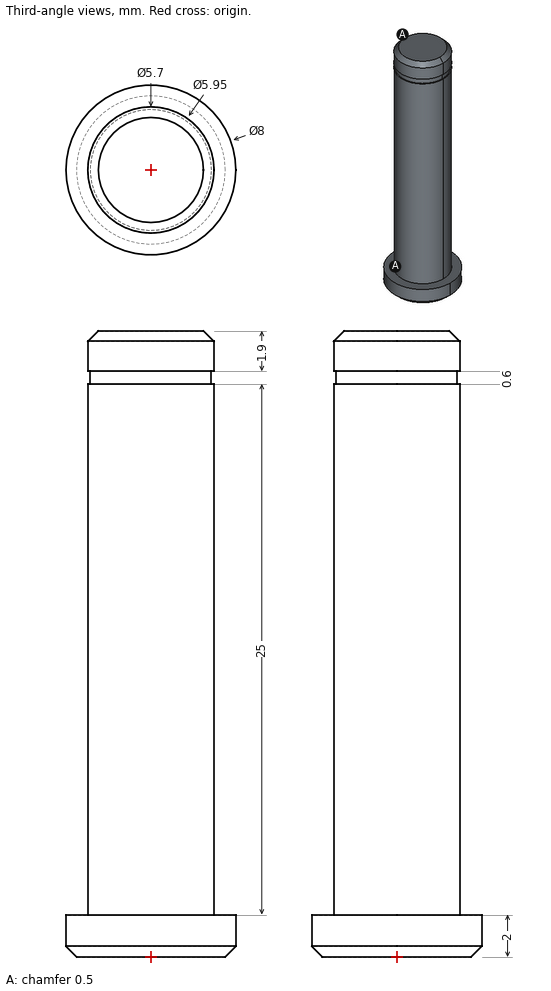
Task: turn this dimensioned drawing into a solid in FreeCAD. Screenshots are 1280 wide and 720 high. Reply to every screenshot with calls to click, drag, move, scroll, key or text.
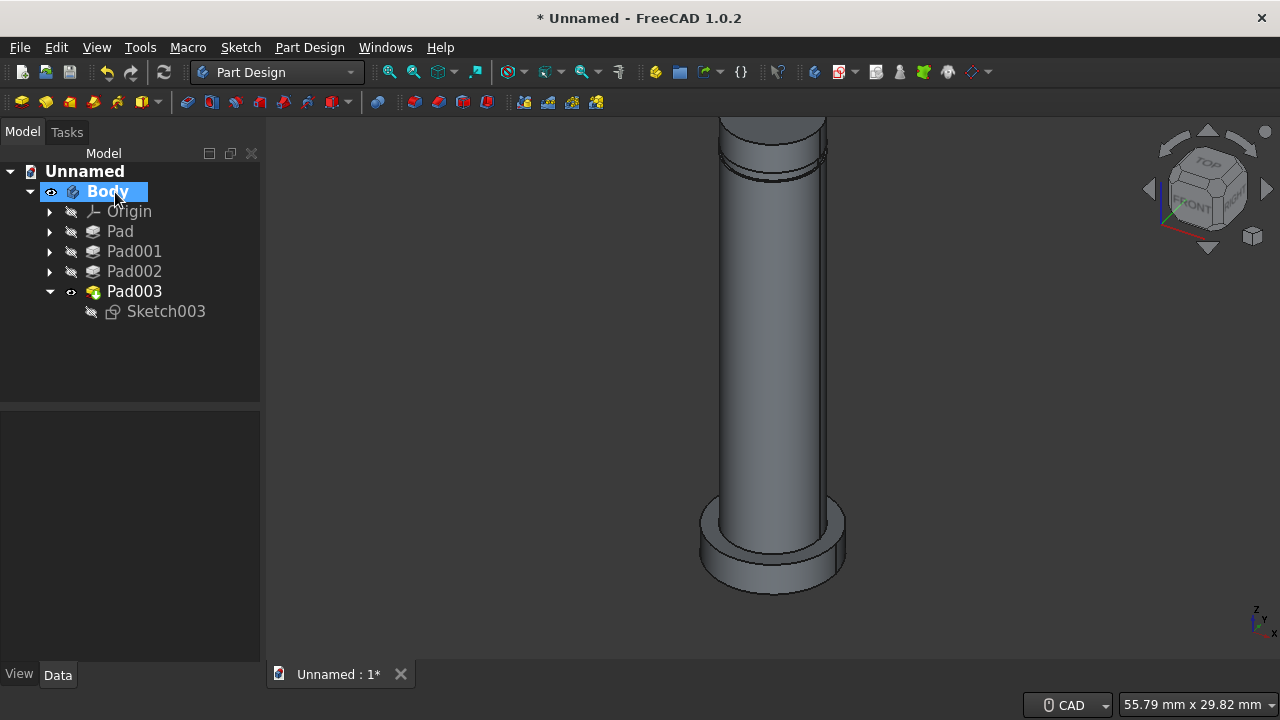
key(v)
key(f)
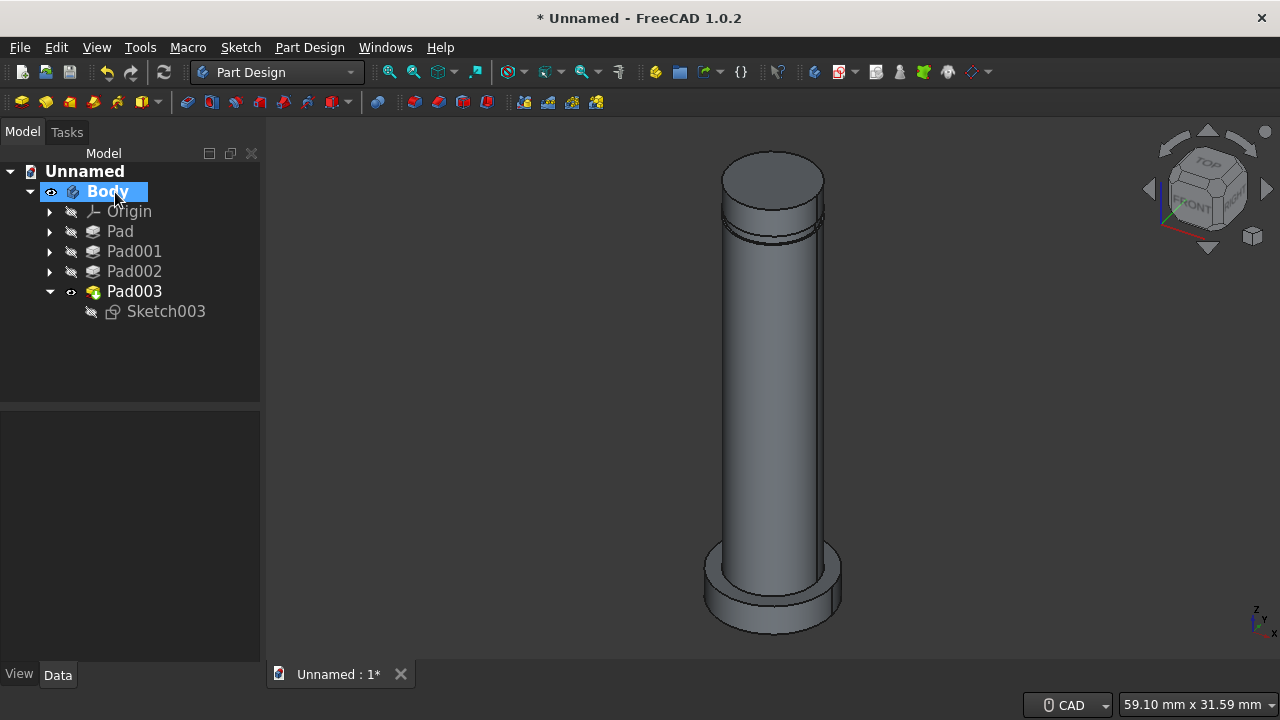
click(722, 183)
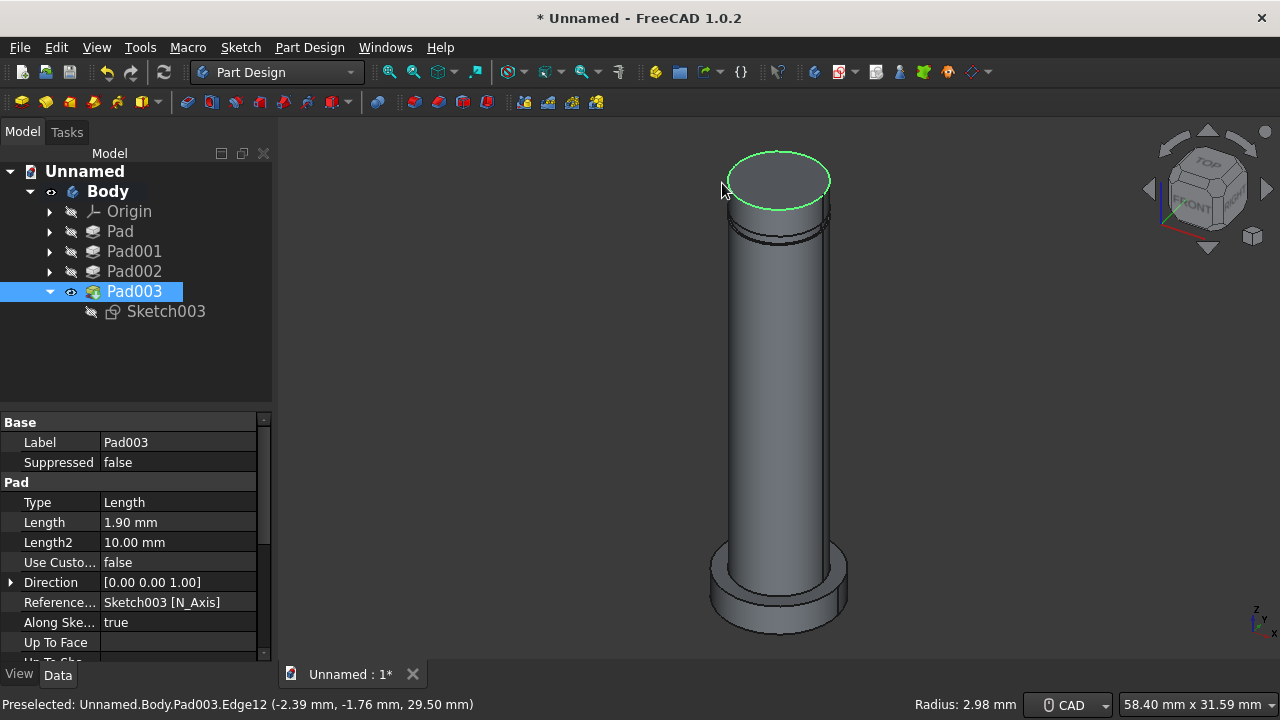
key(0)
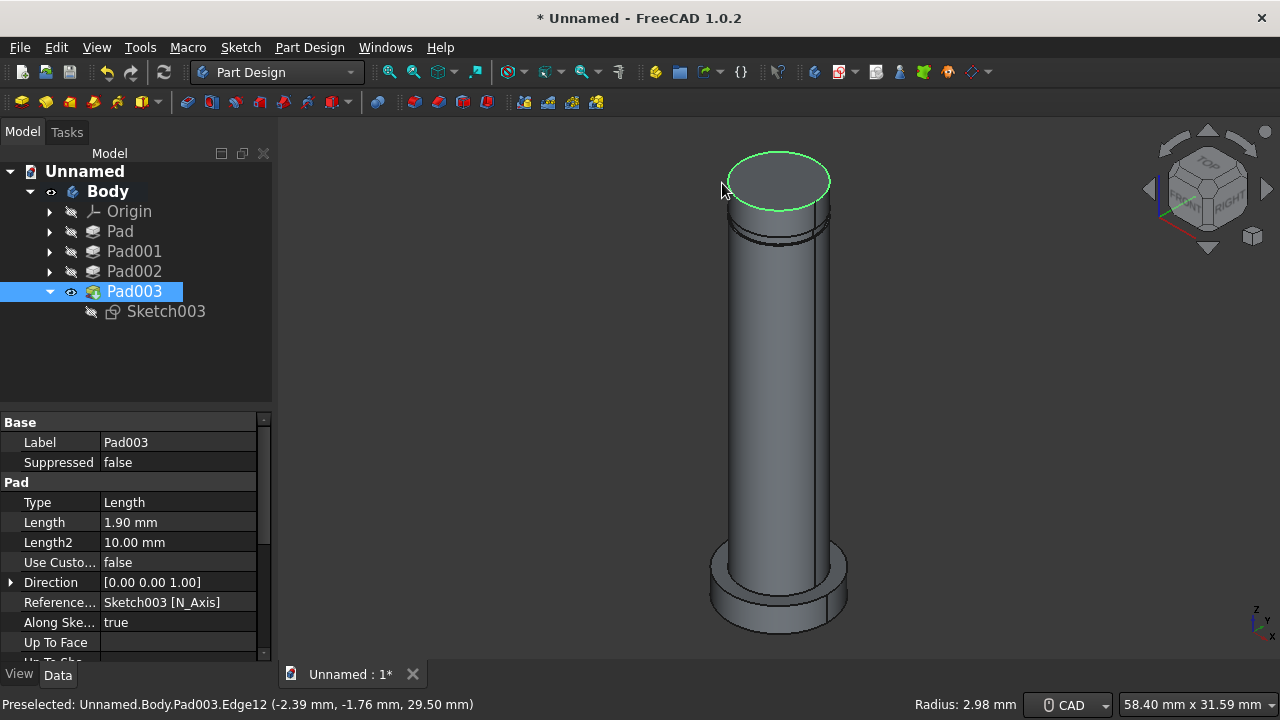
key(2)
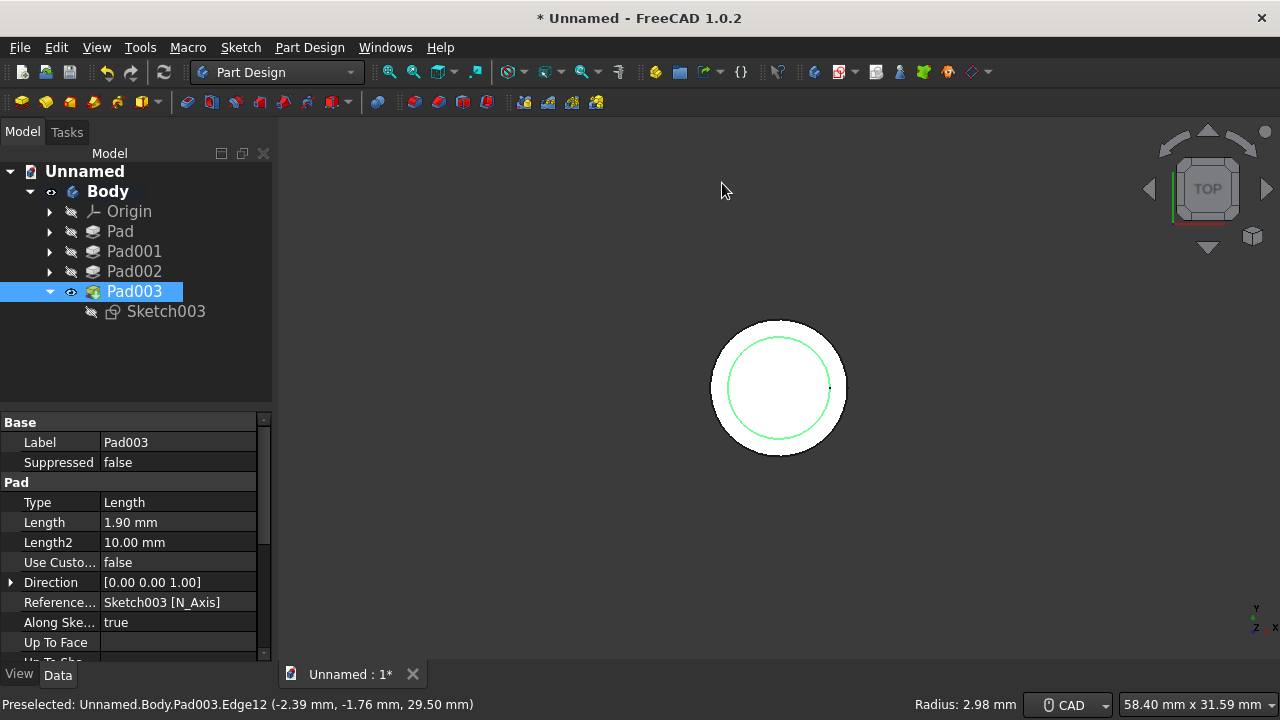
click(390, 72)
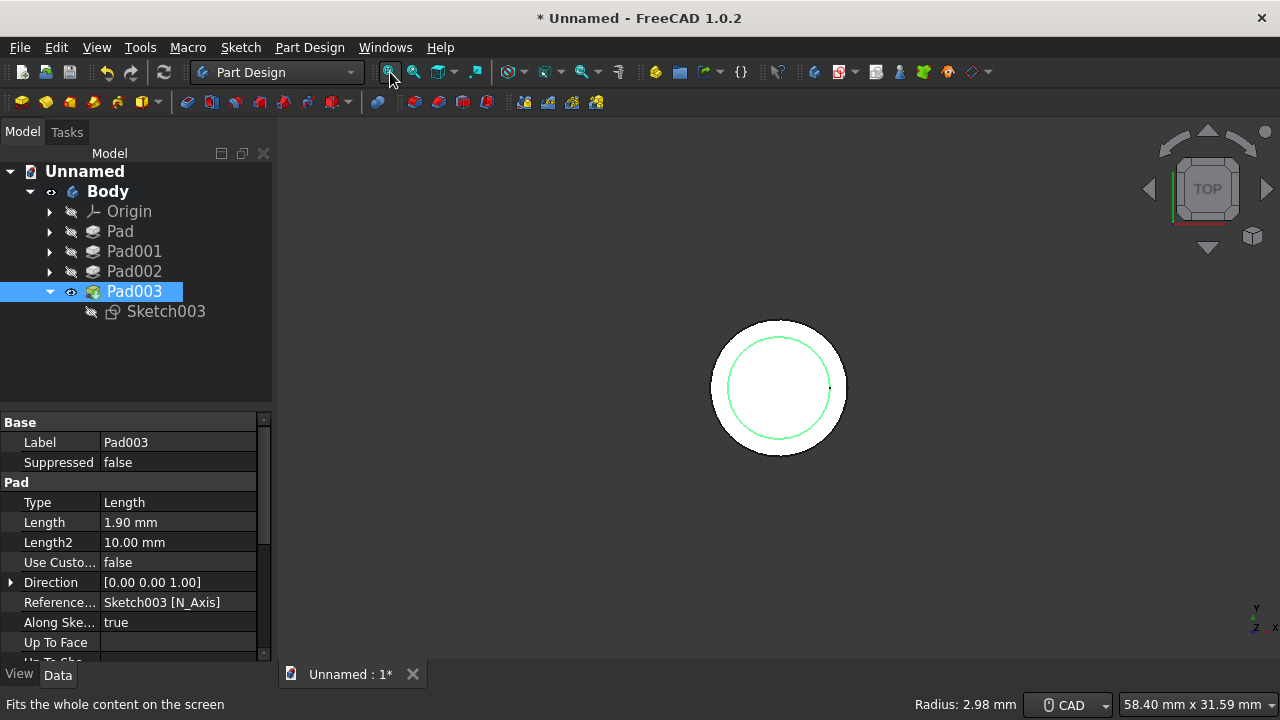
key(1)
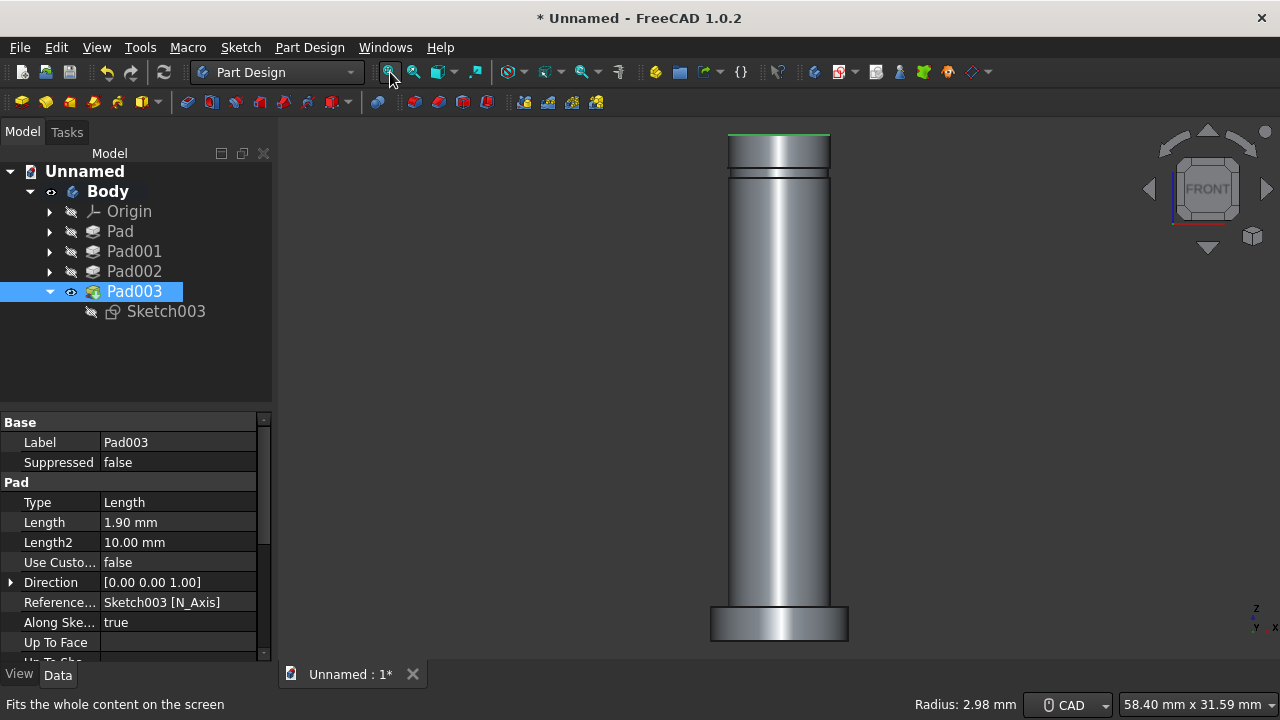
key(3)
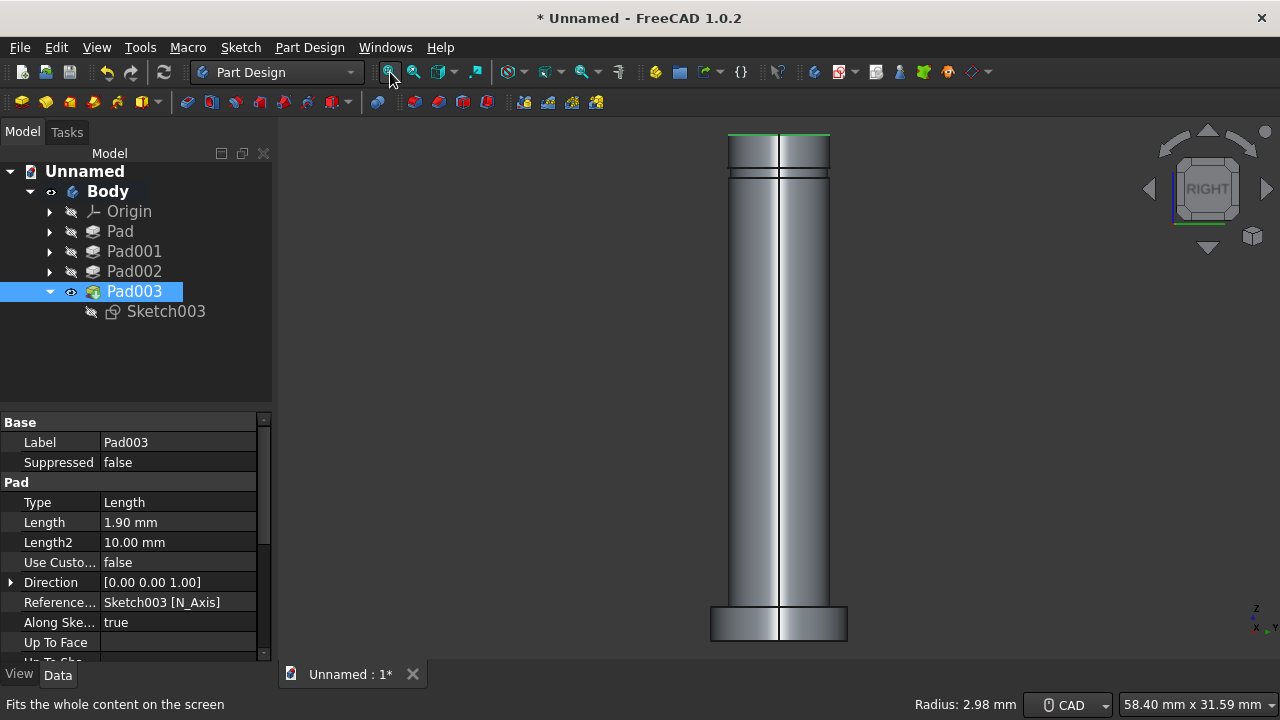
key(5)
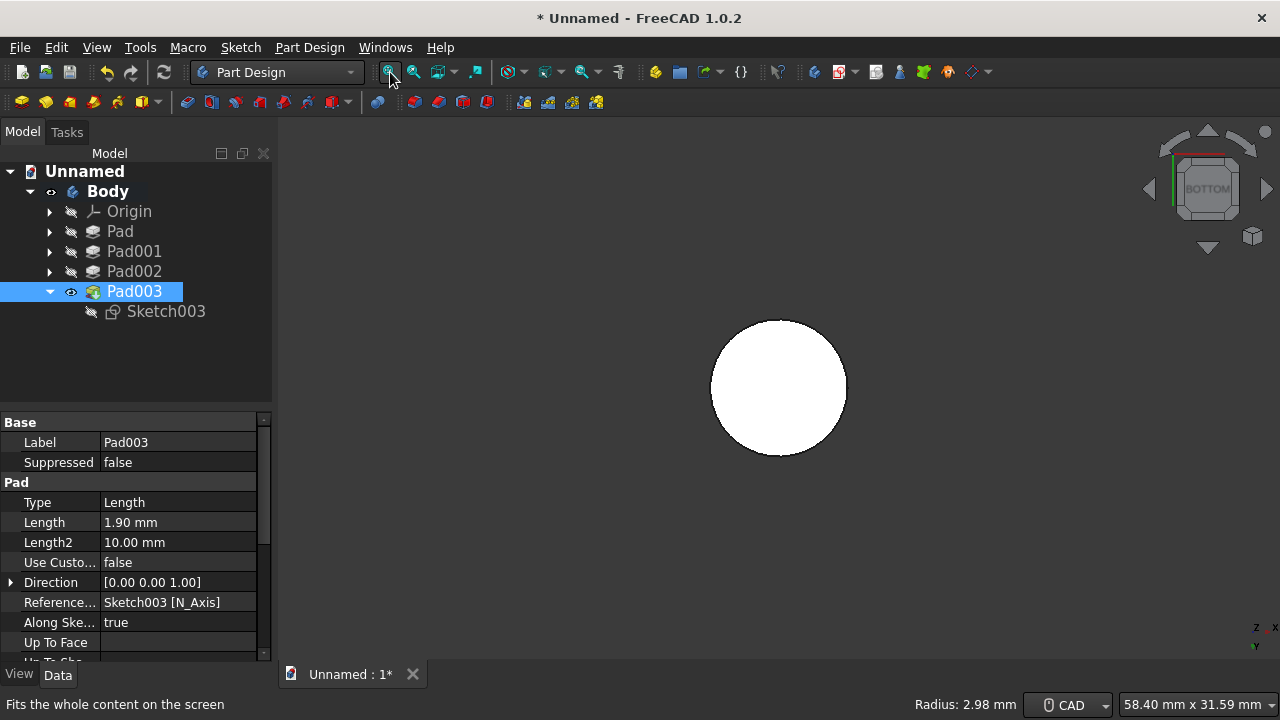
key(v)
key(f)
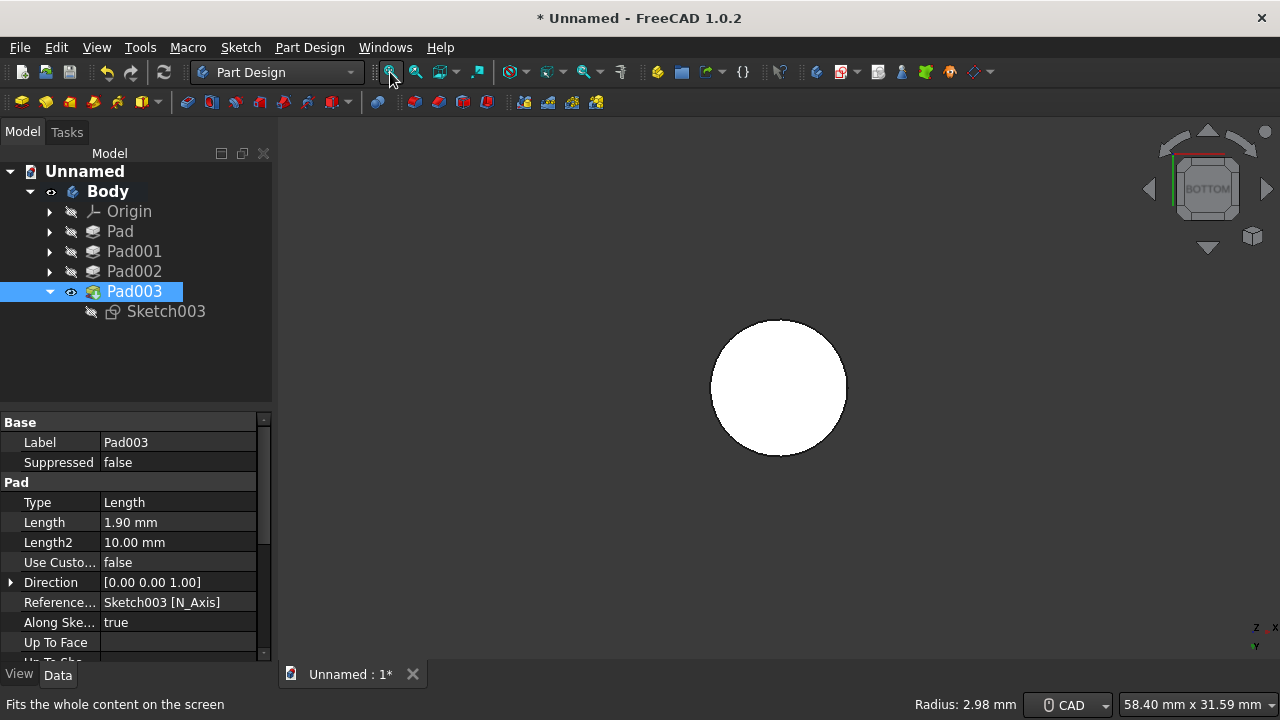
click(710, 387, ctrl)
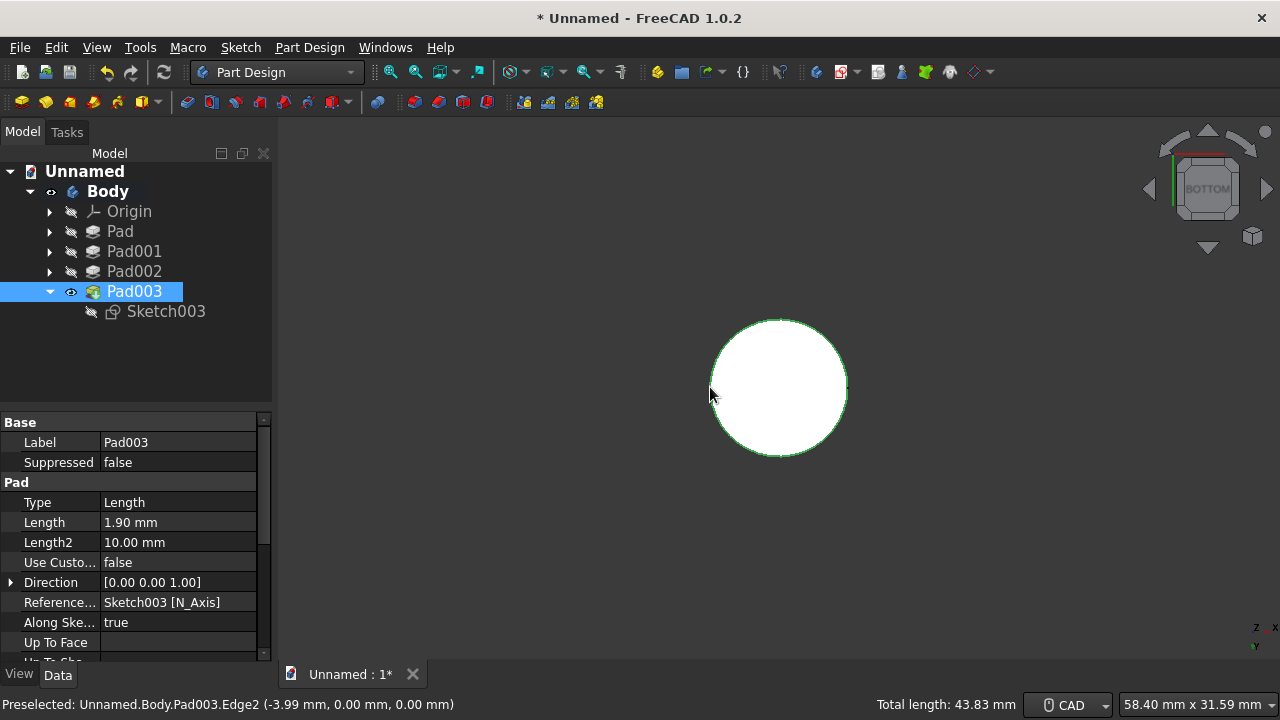
click(440, 102)